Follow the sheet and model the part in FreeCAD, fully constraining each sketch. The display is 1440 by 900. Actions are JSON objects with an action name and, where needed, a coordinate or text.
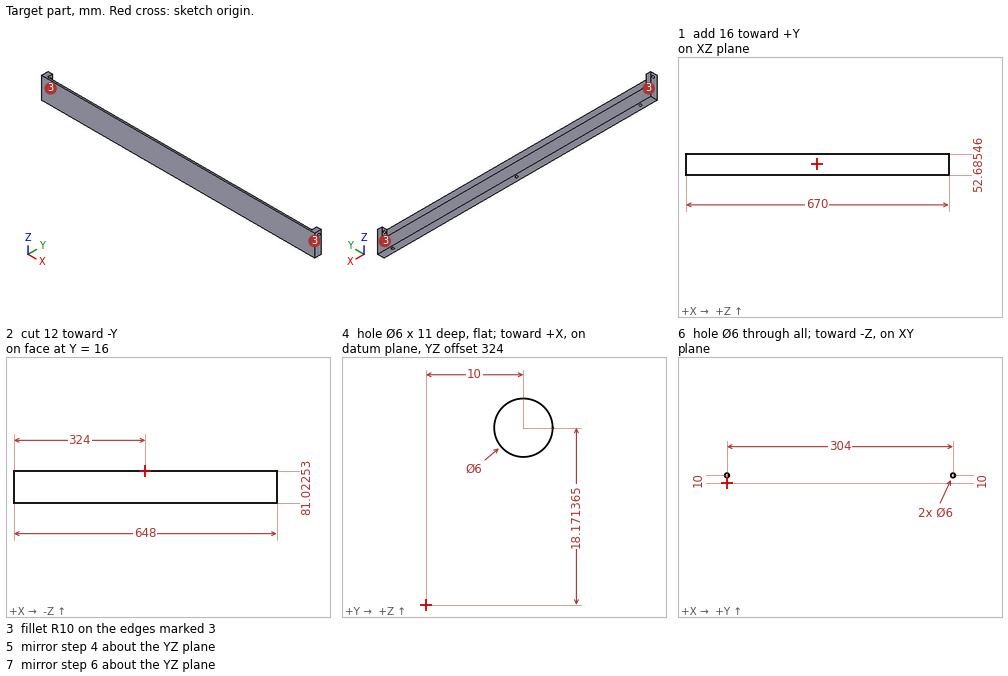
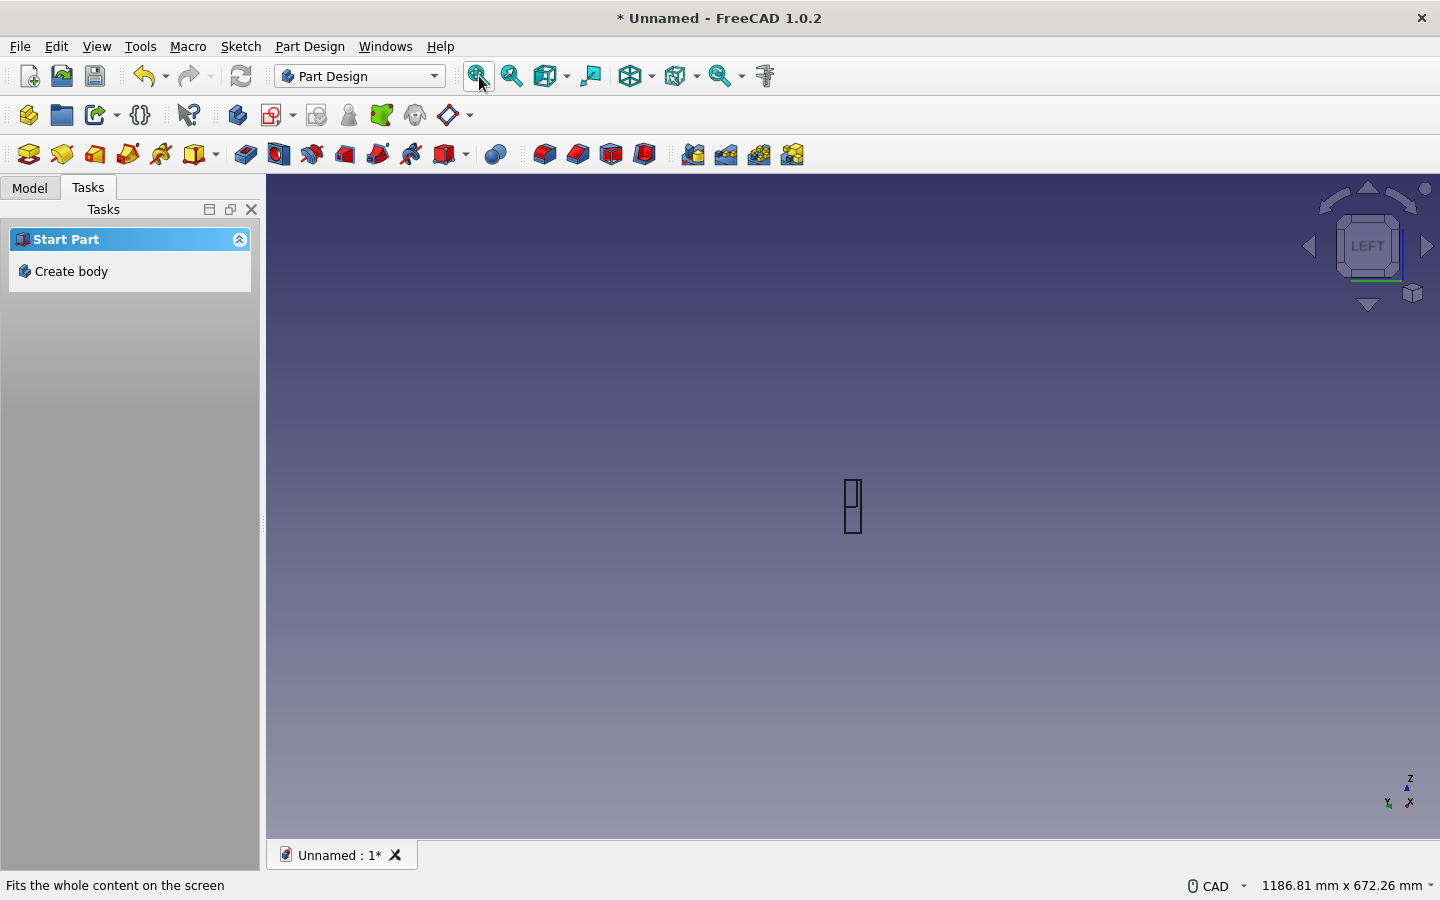
{"action": "key", "text": "0"}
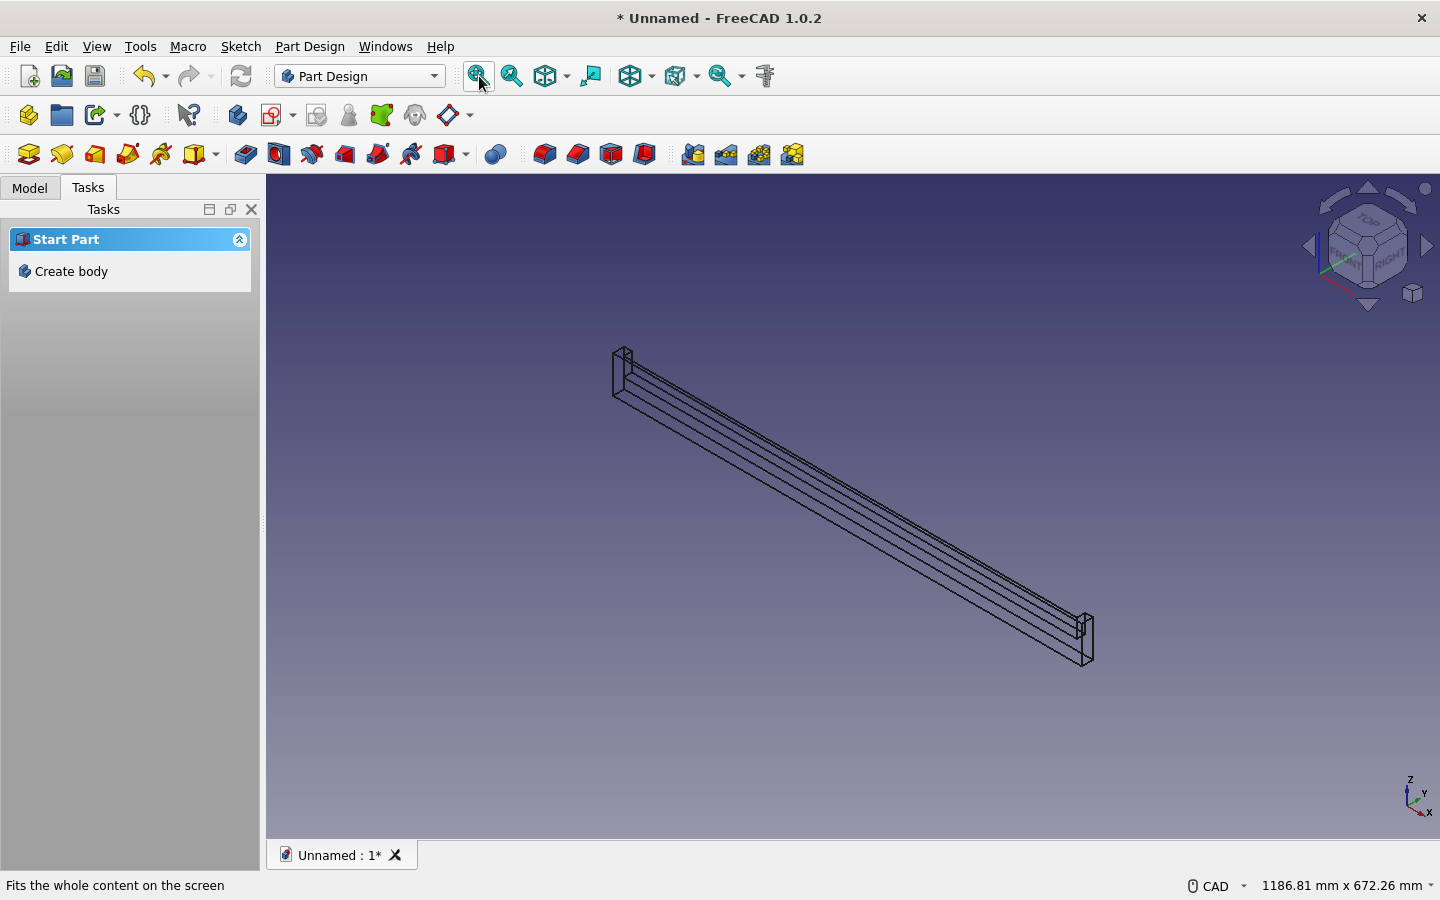
{"action": "left_click", "coordinate": [630, 372]}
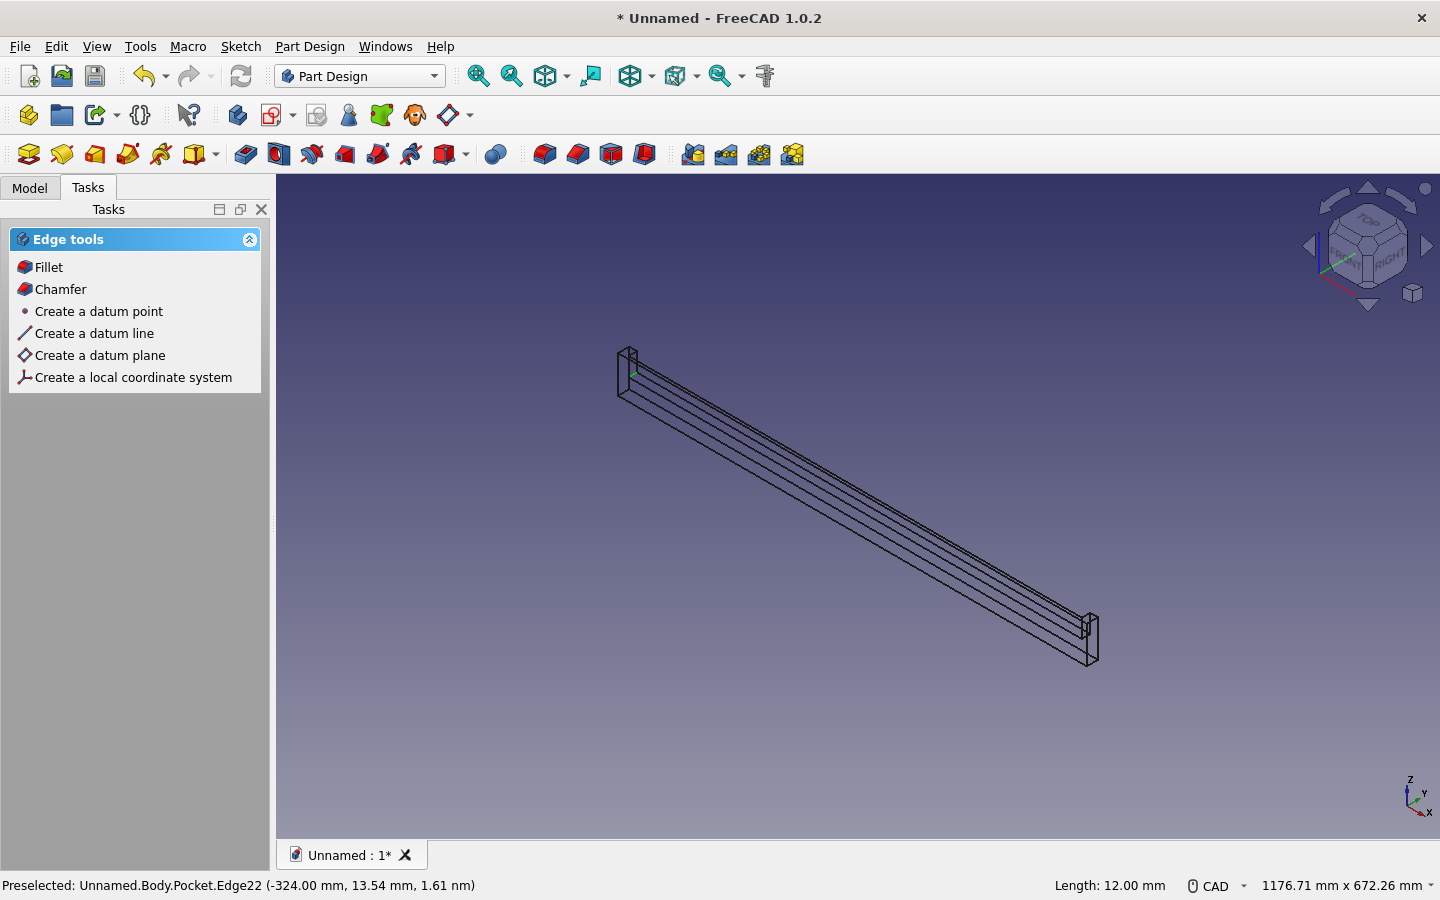
{"action": "scroll", "coordinate": [1086, 636], "scroll_direction": "up", "scroll_amount": 7}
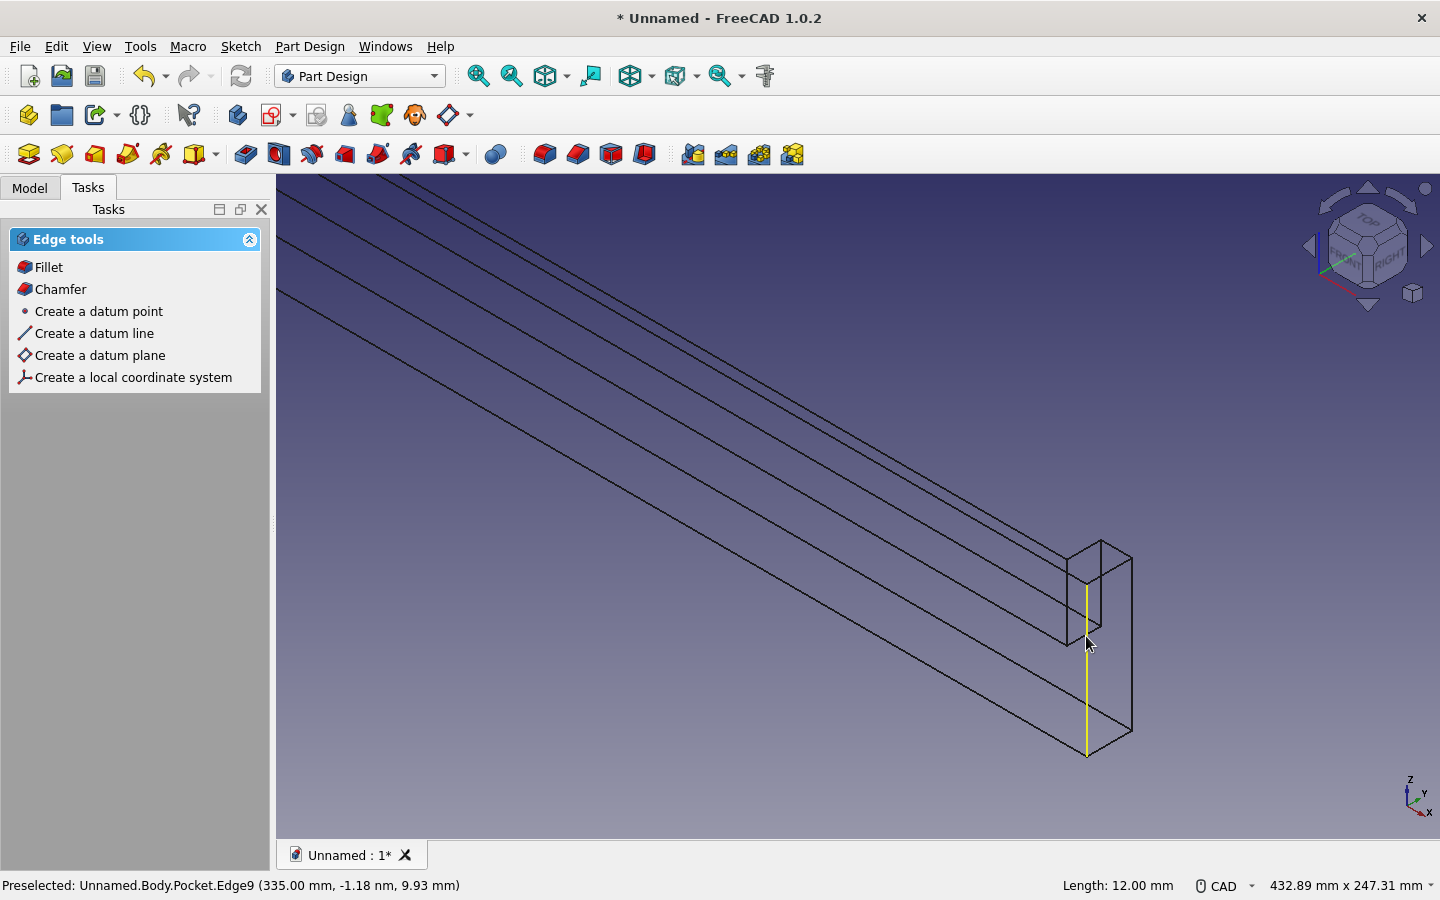
{"action": "left_click", "coordinate": [1077, 639], "text": "ctrl"}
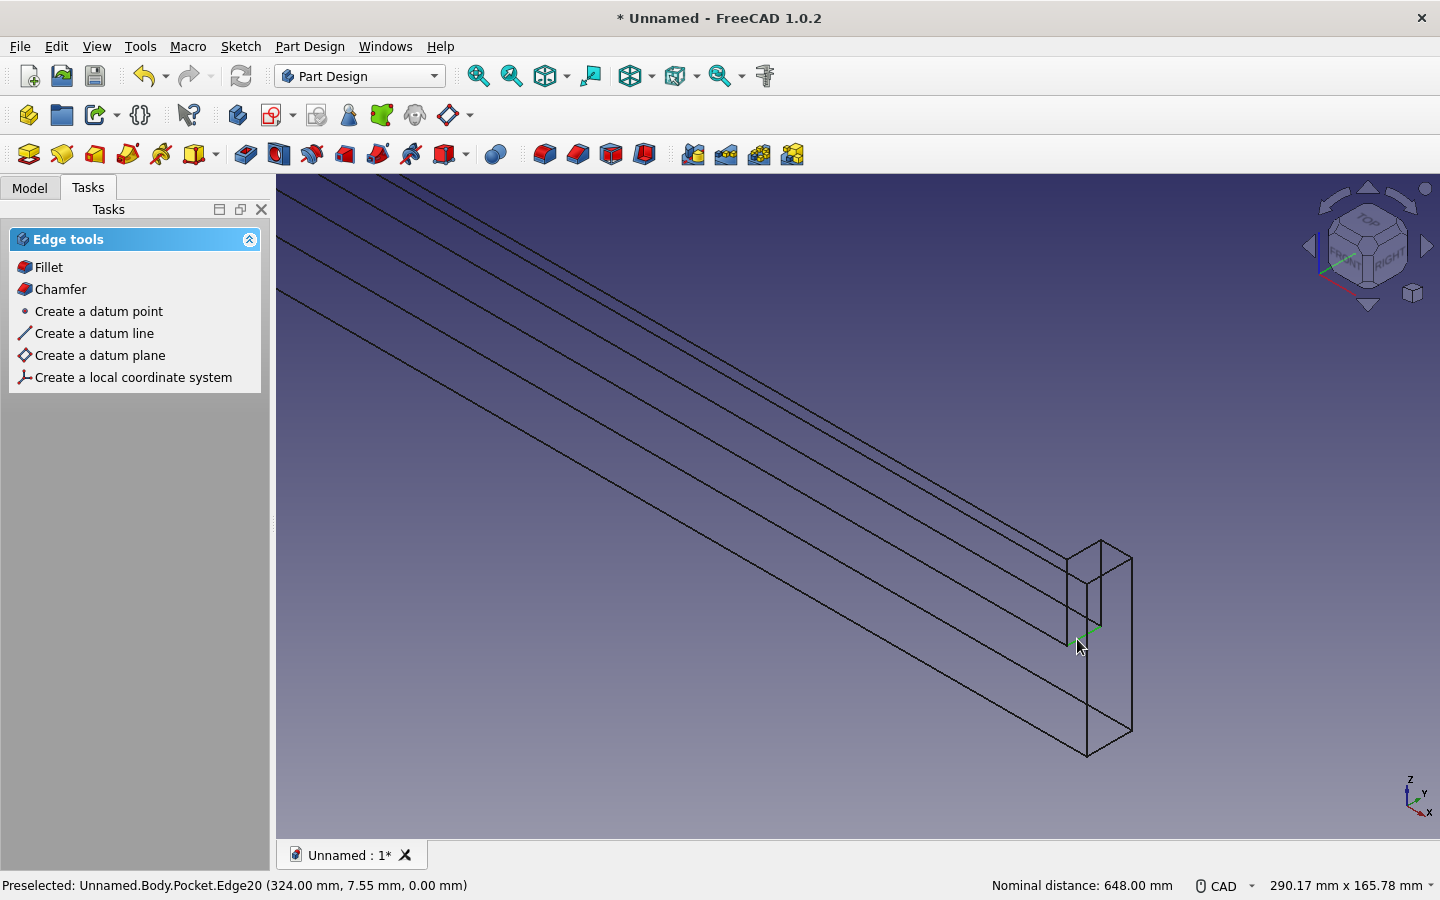
{"action": "key", "text": "v 1"}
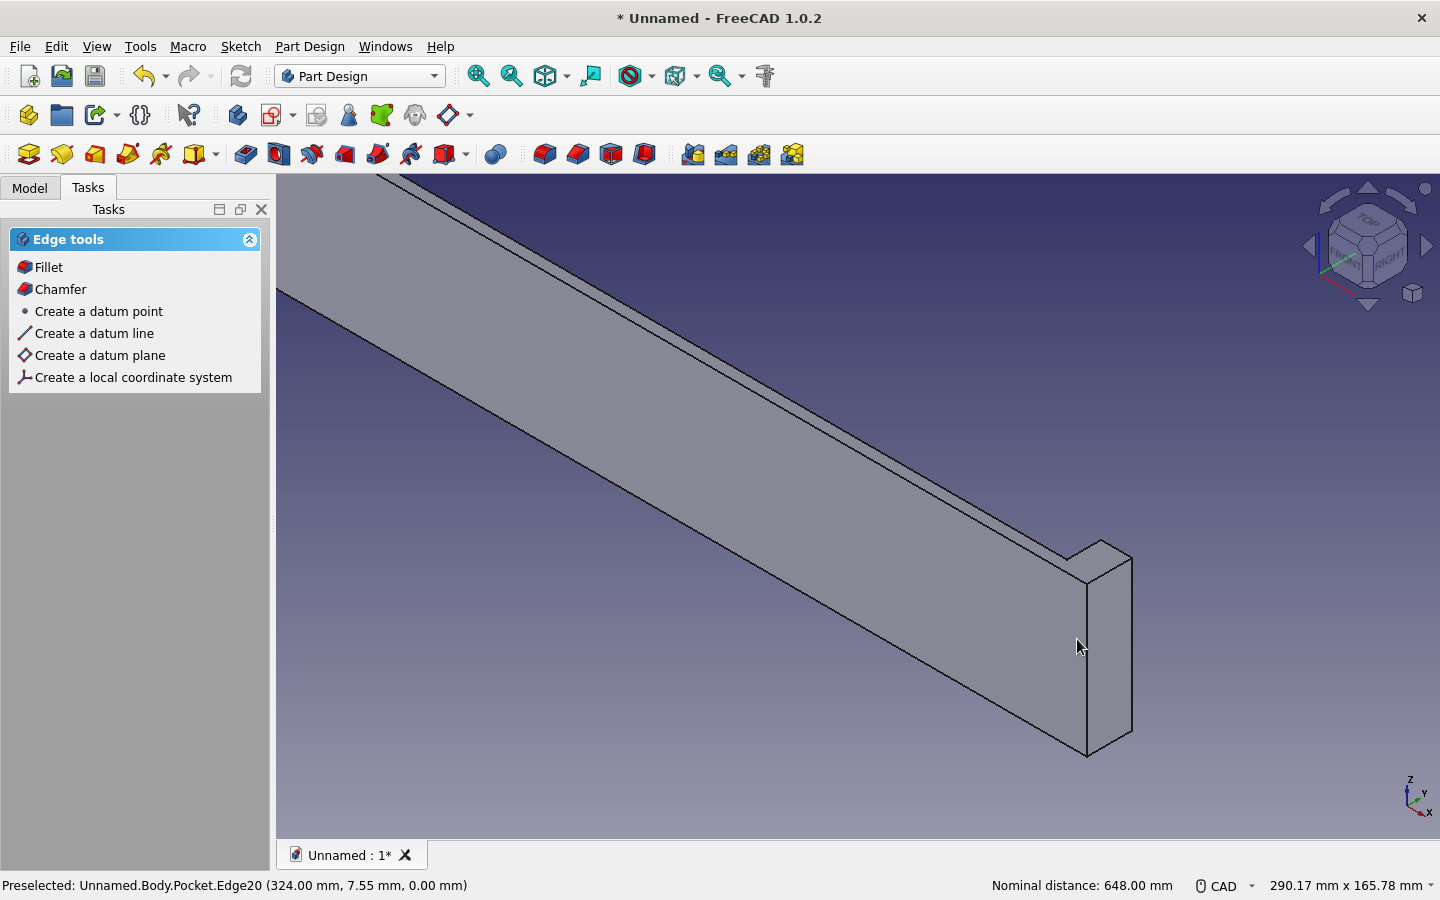
{"action": "left_click", "coordinate": [545, 154]}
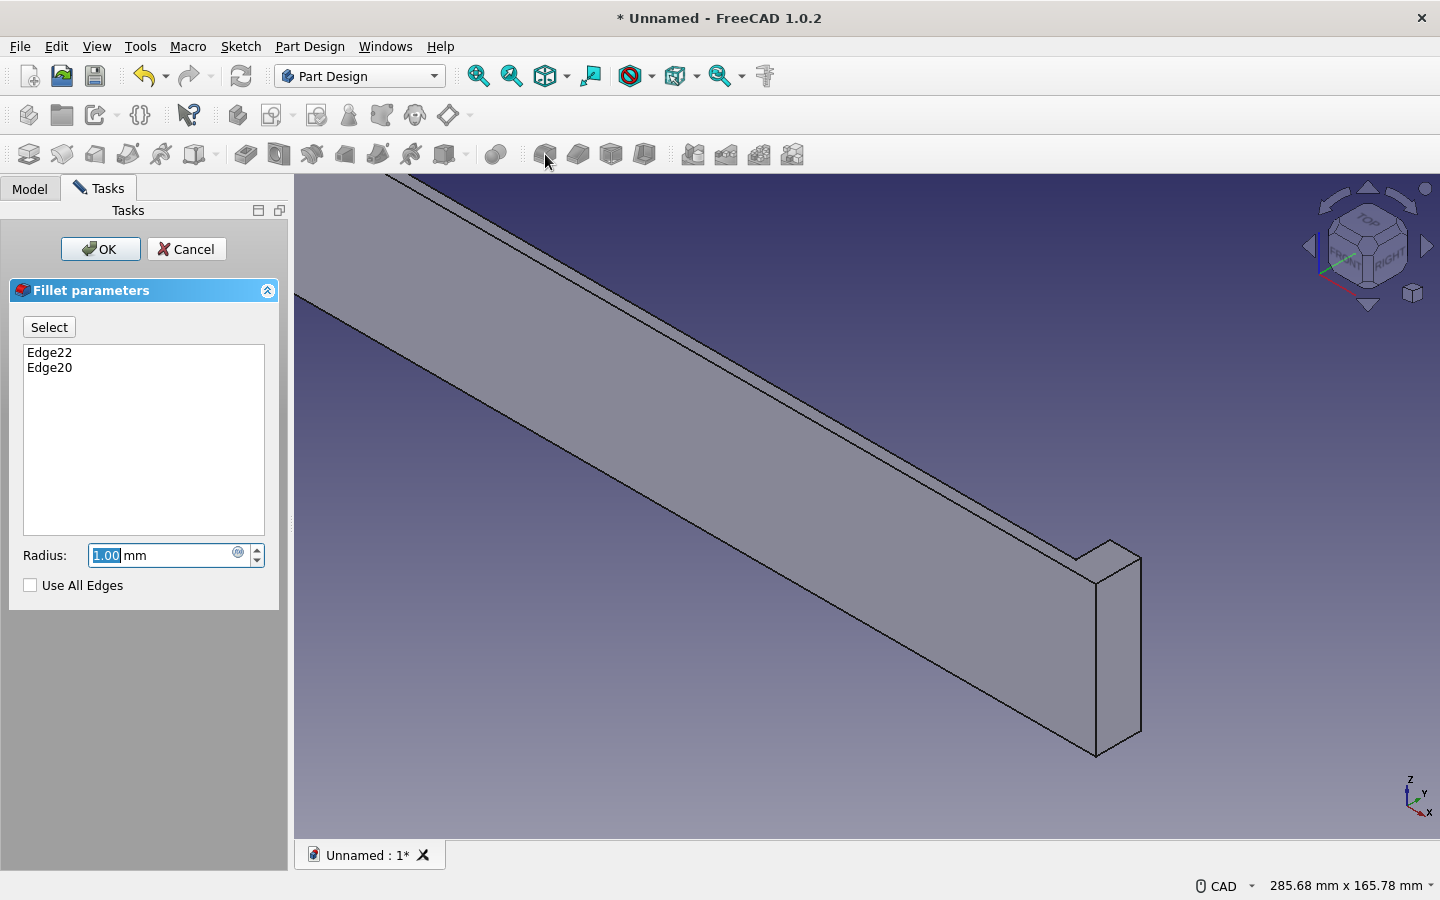
{"action": "type", "text": "10"}
{"action": "key", "text": "Tab"}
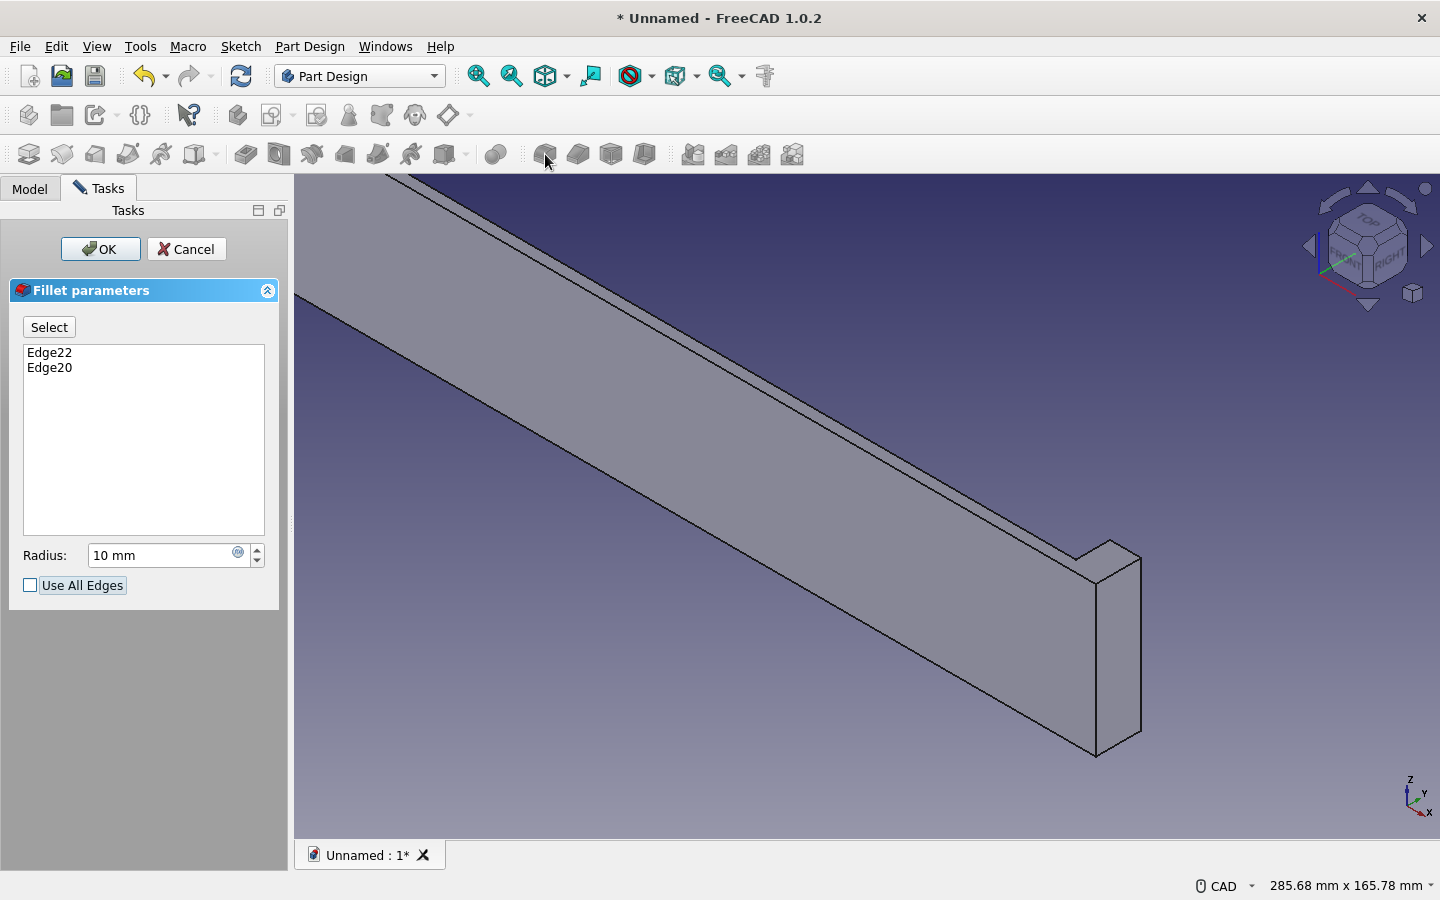
{"action": "left_click", "coordinate": [101, 249]}